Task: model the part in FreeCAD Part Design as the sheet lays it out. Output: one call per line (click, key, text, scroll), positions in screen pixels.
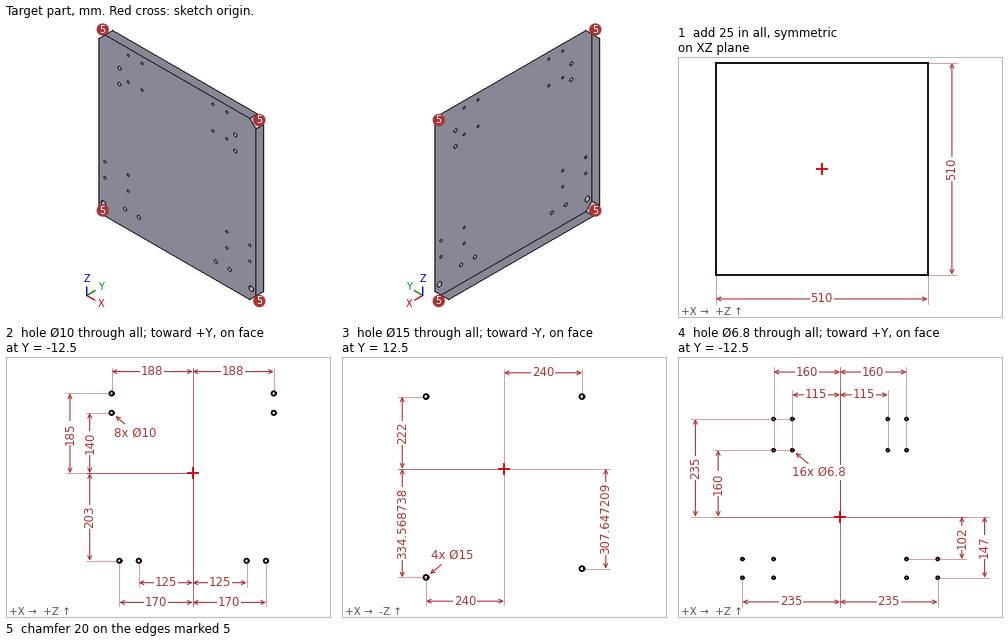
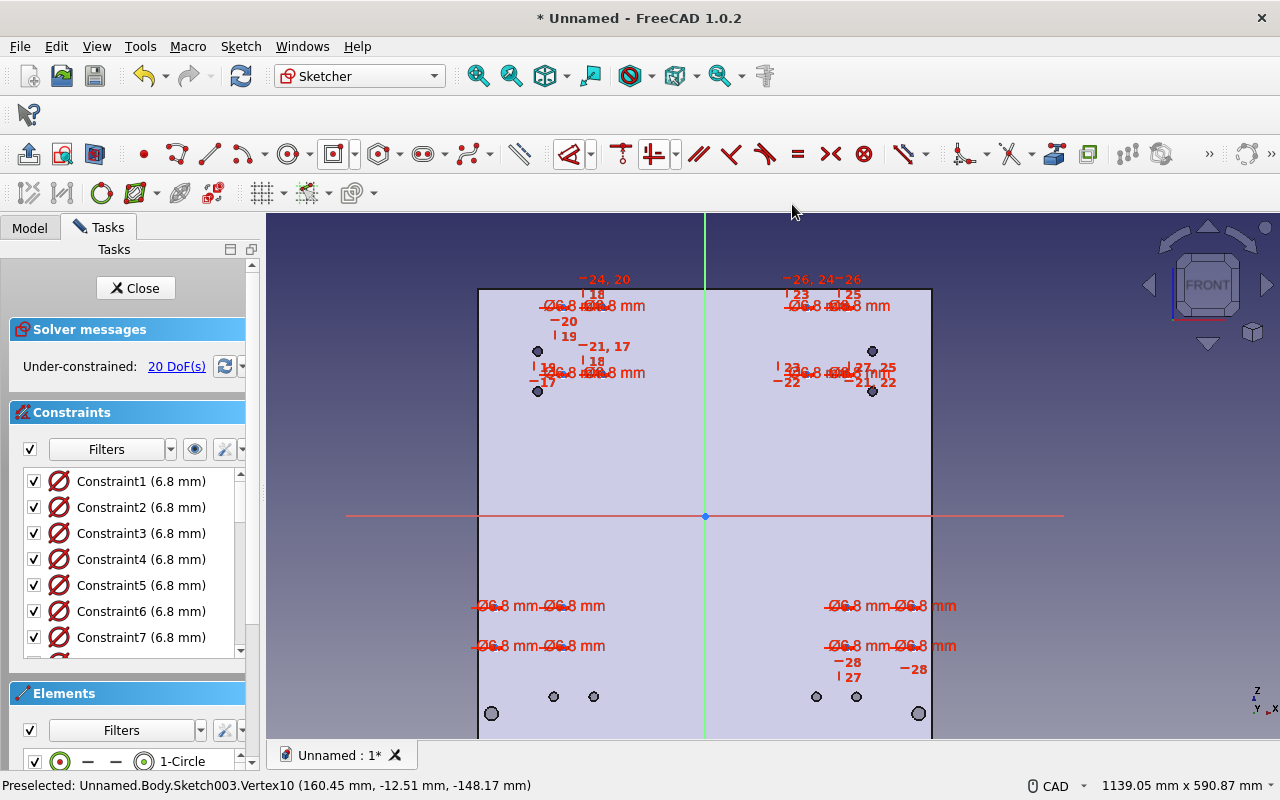
click(848, 648)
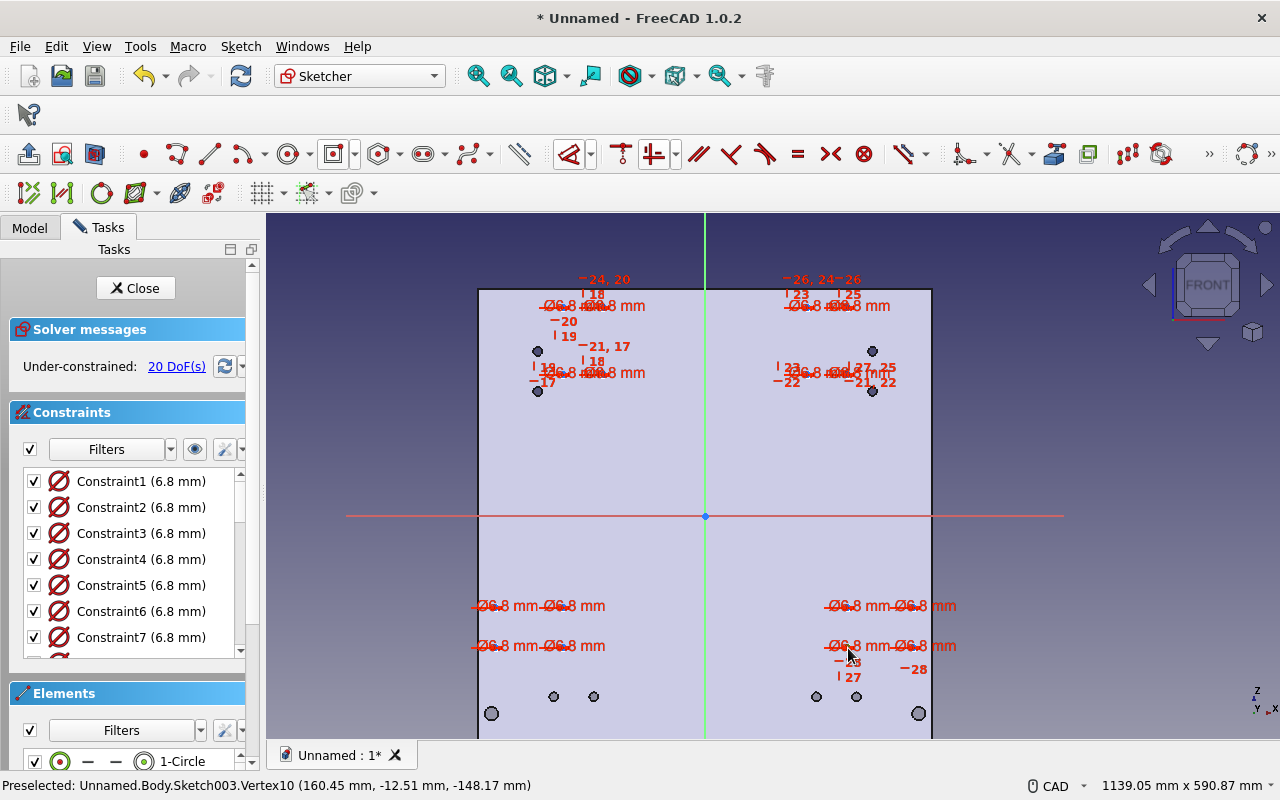
click(848, 608)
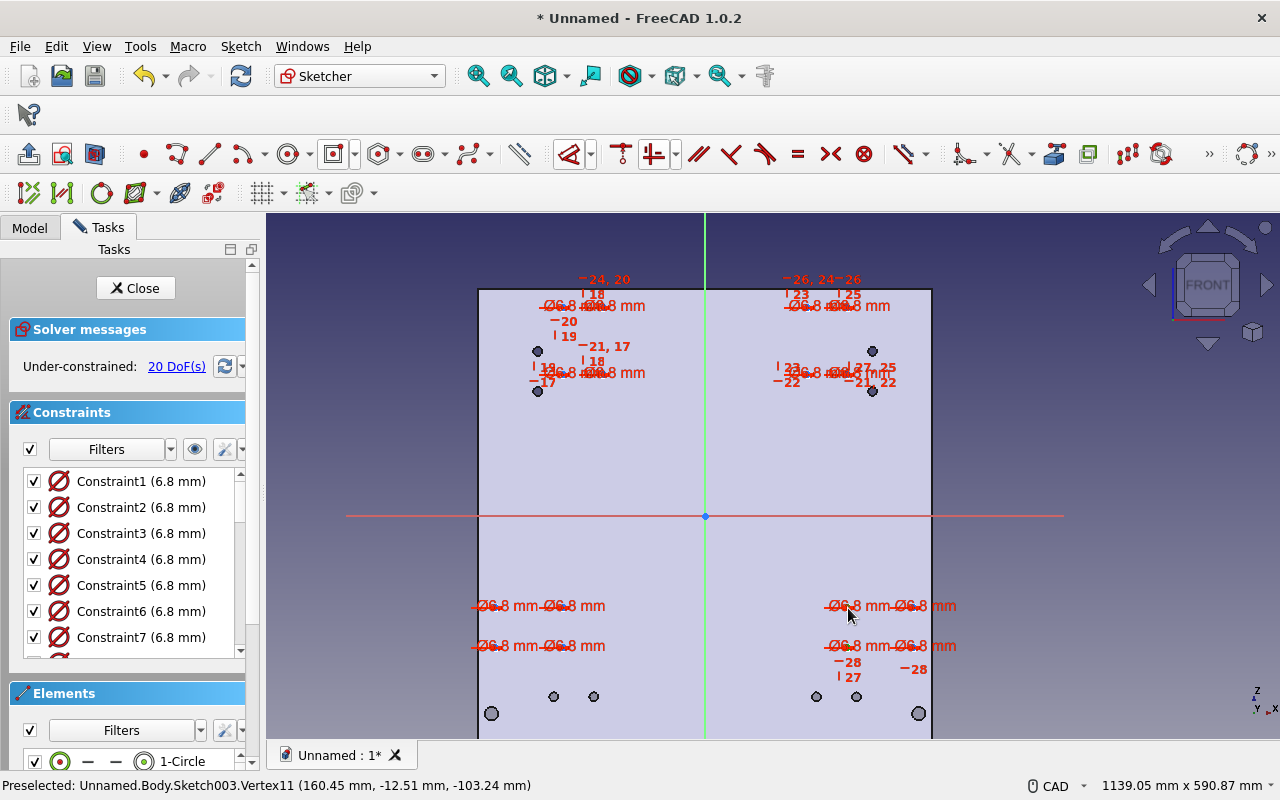
key(v)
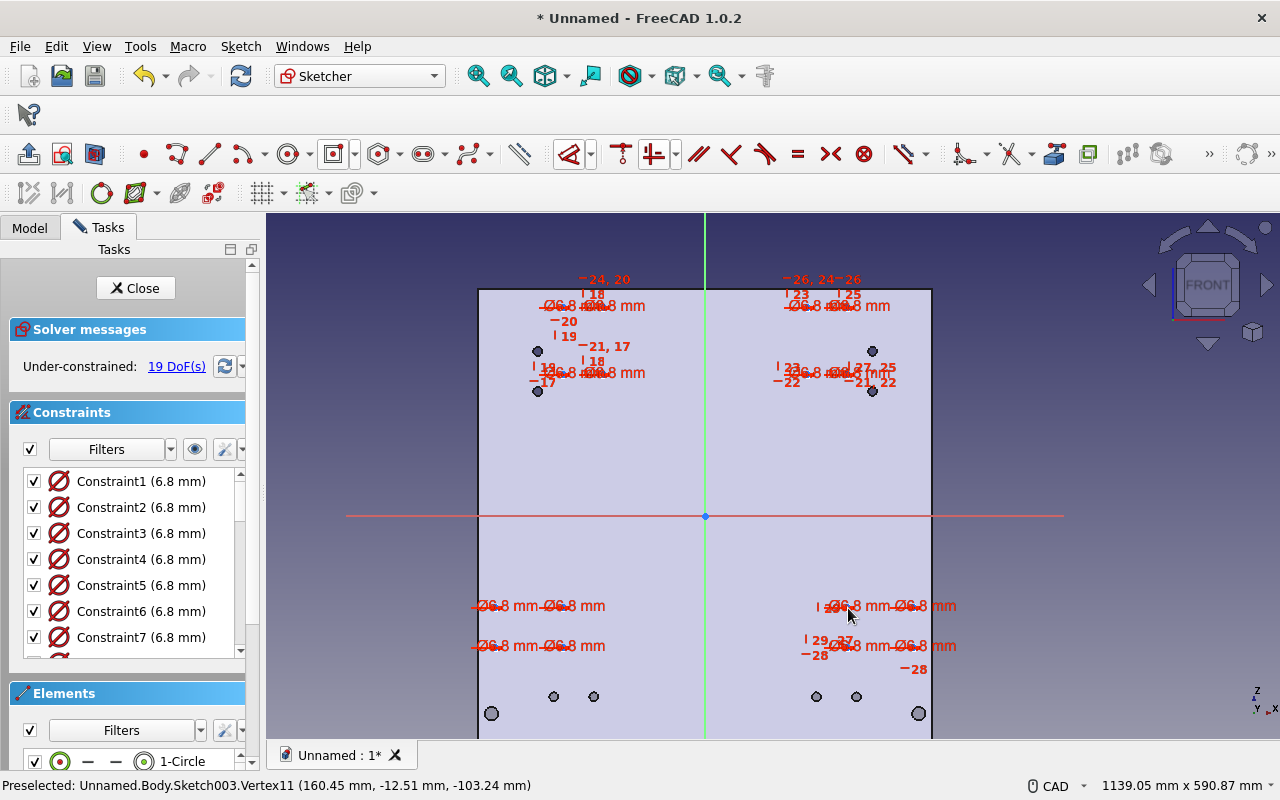
click(914, 648)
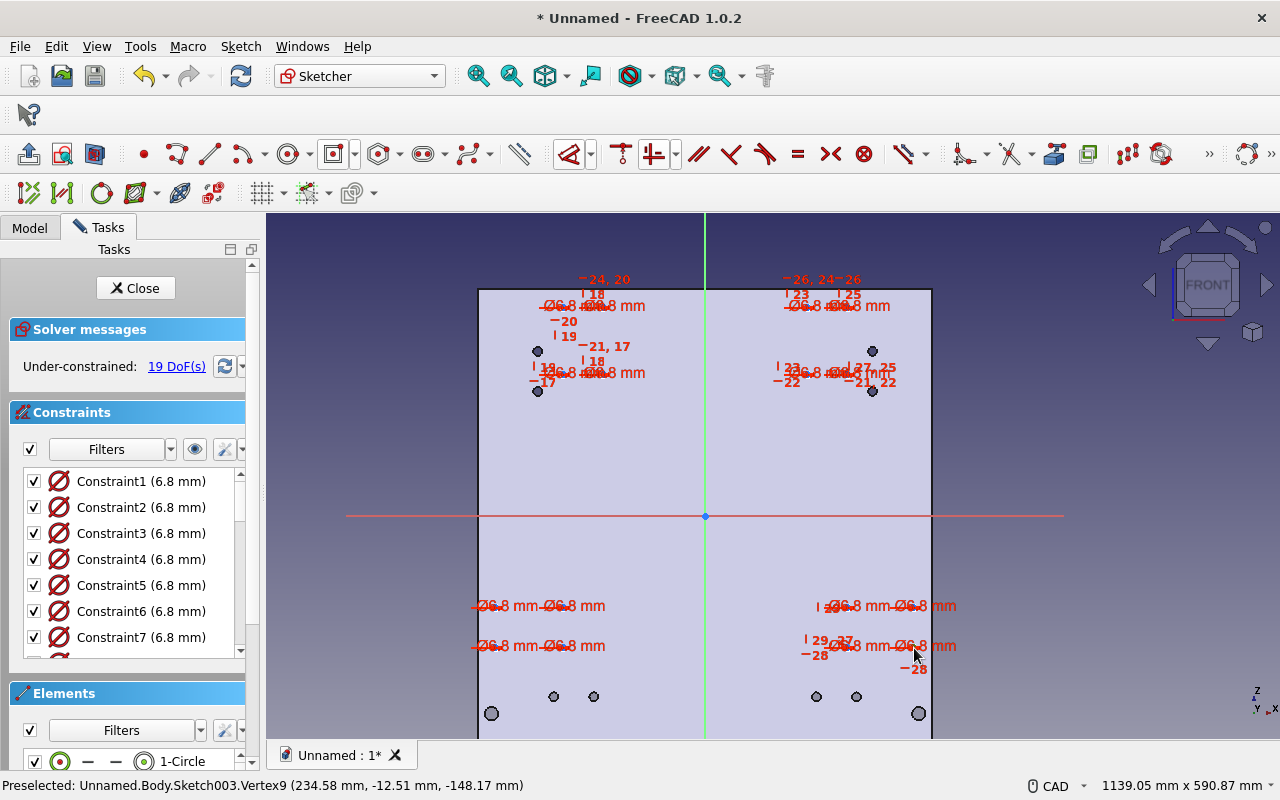
click(914, 608)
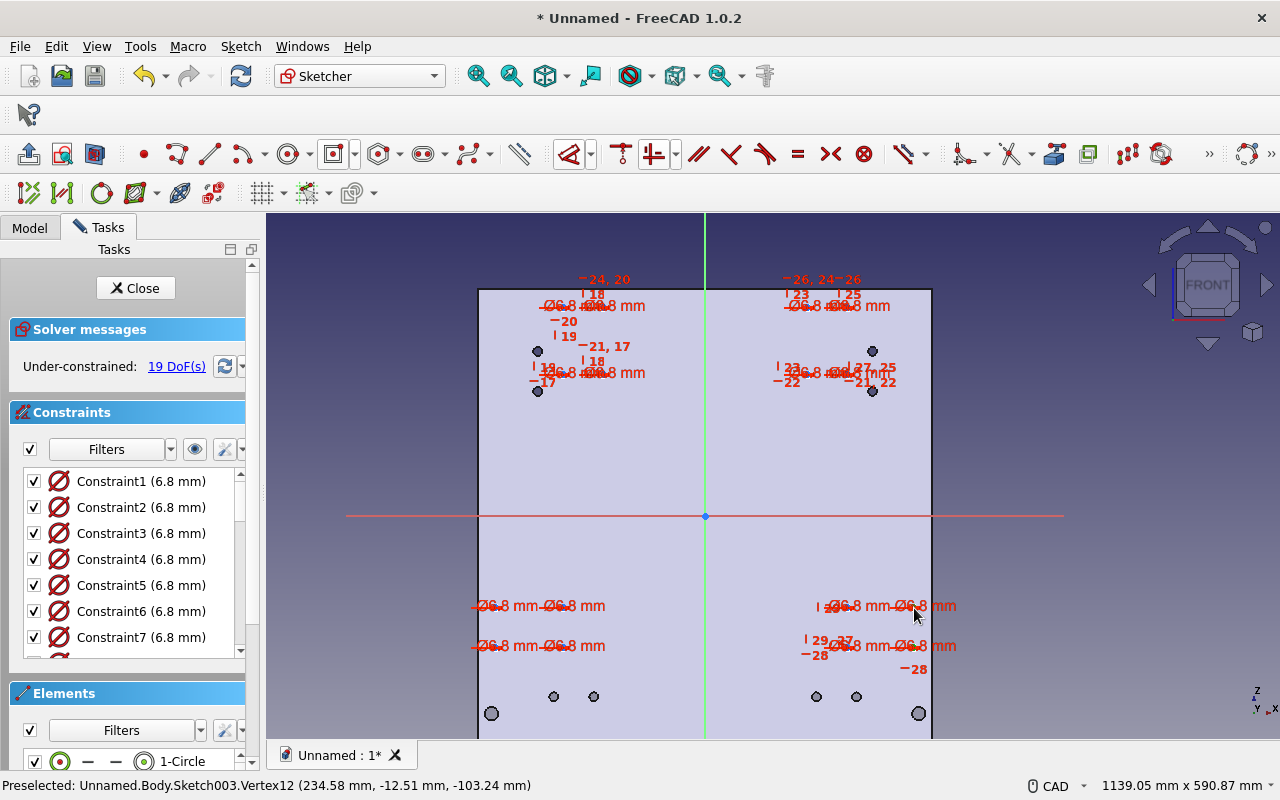
key(v)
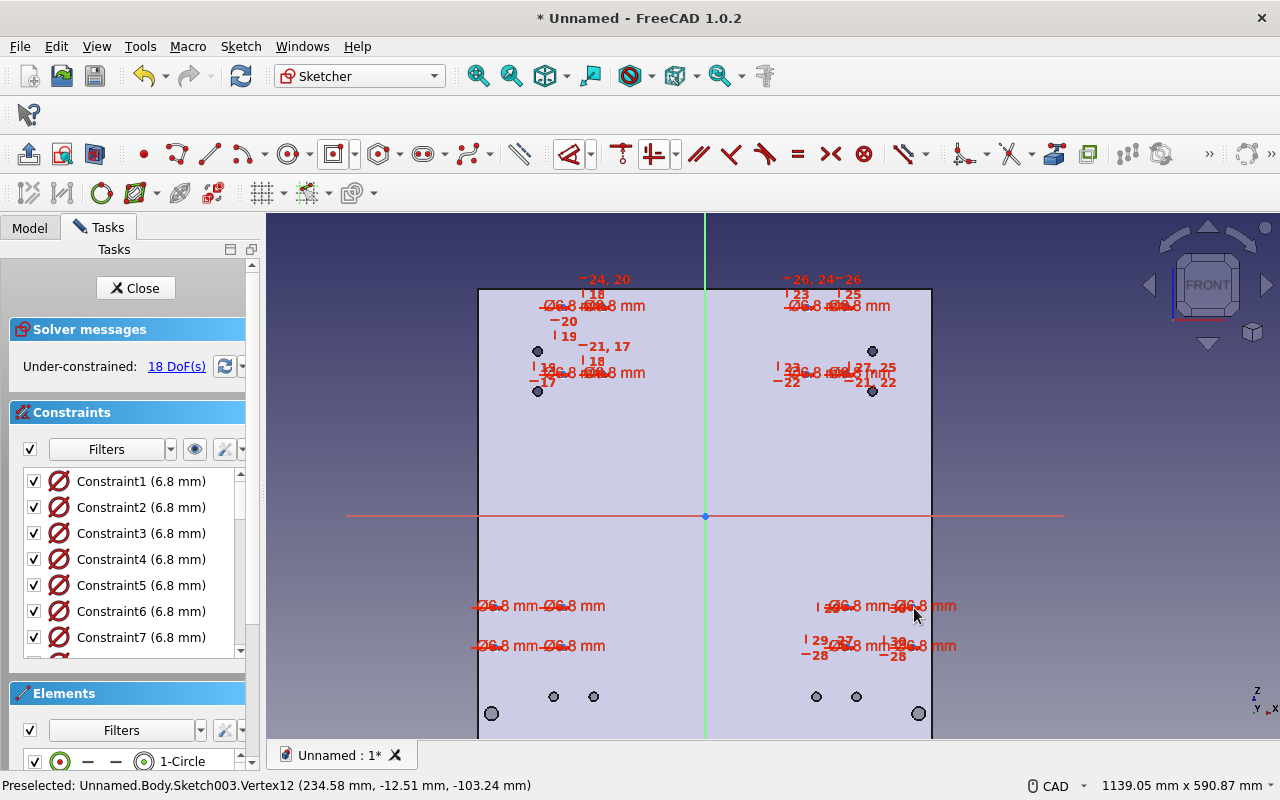
click(848, 608)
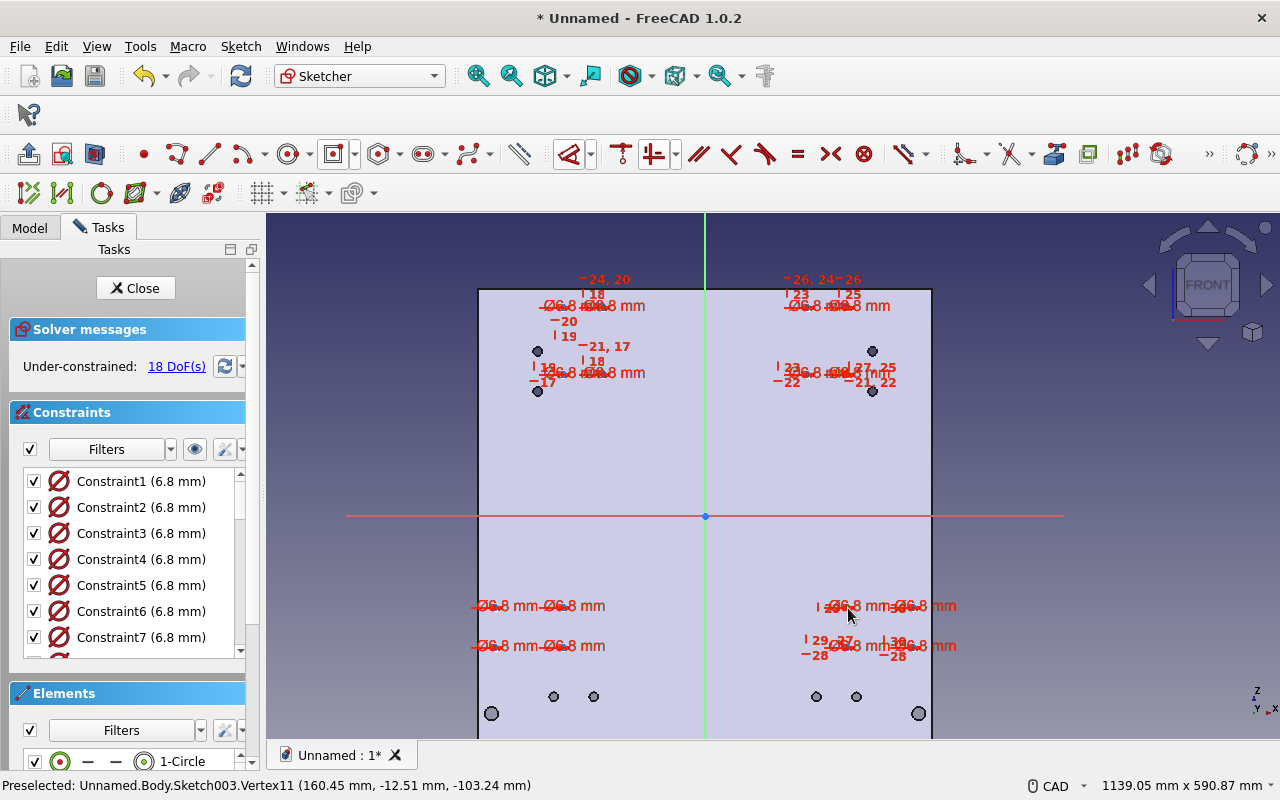
click(914, 608)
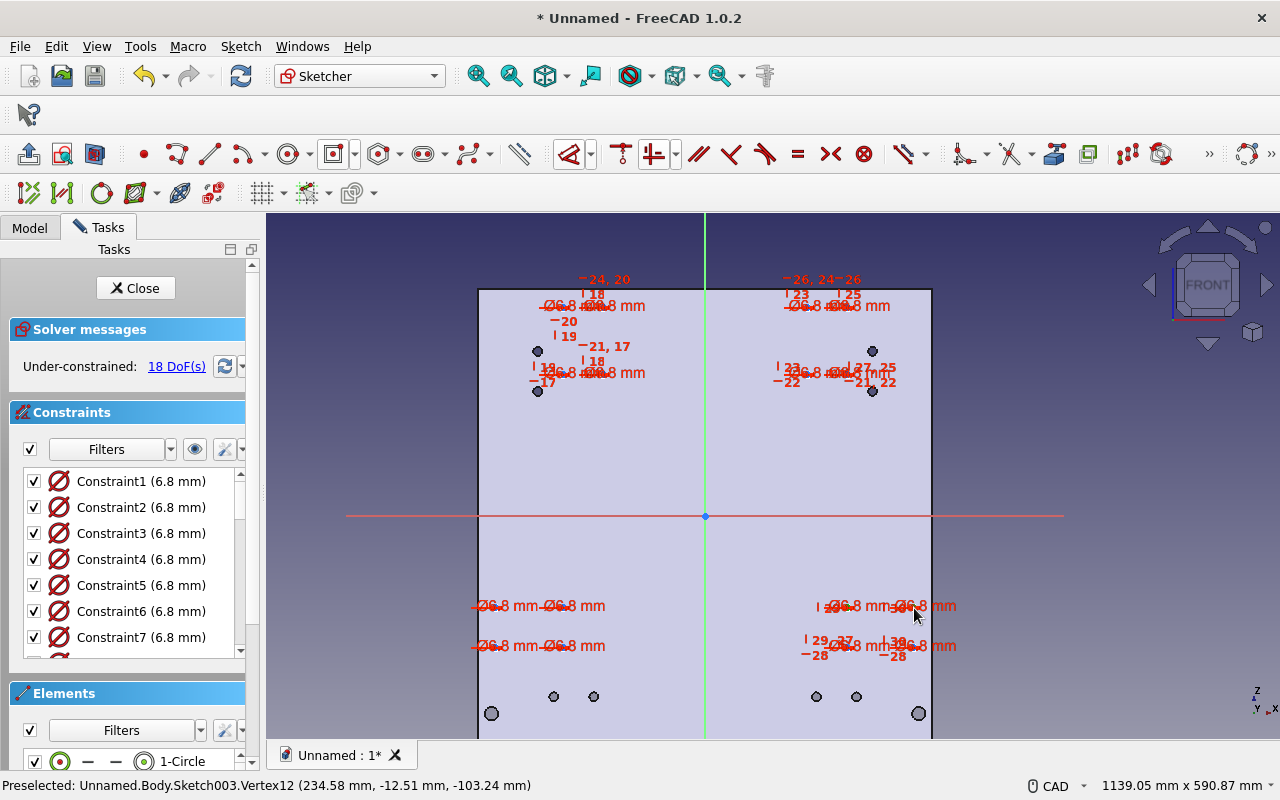
key(h)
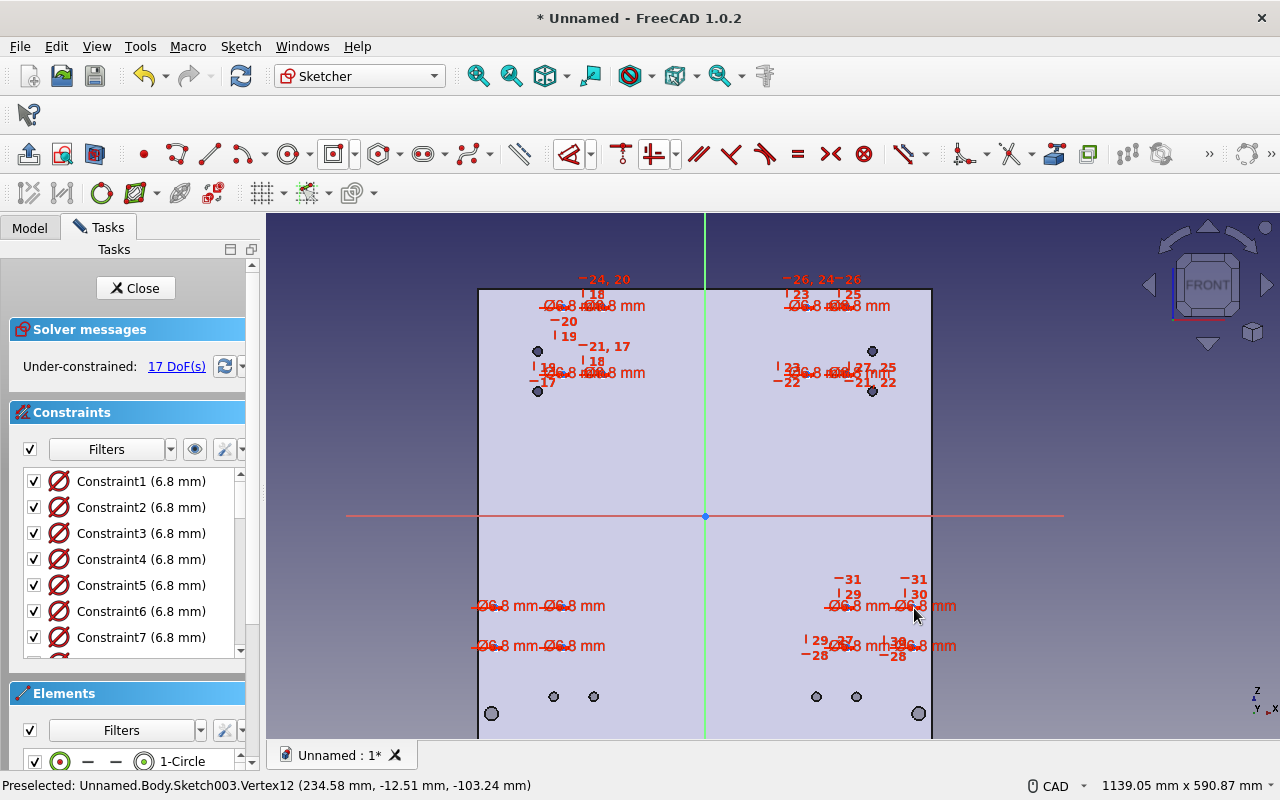
click(563, 375)